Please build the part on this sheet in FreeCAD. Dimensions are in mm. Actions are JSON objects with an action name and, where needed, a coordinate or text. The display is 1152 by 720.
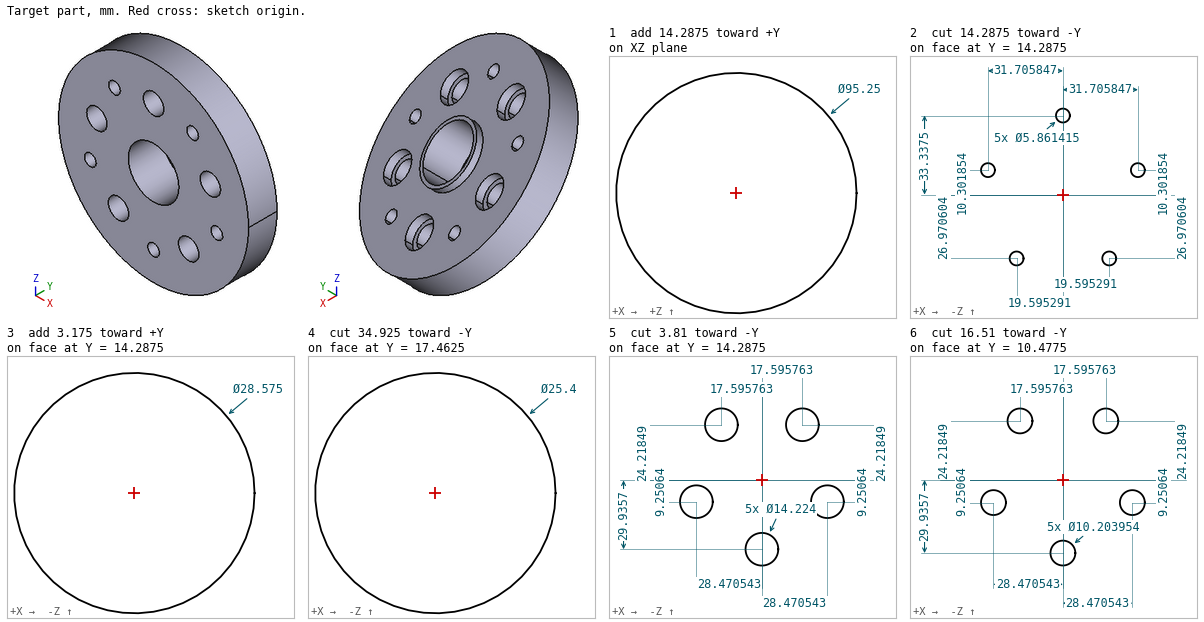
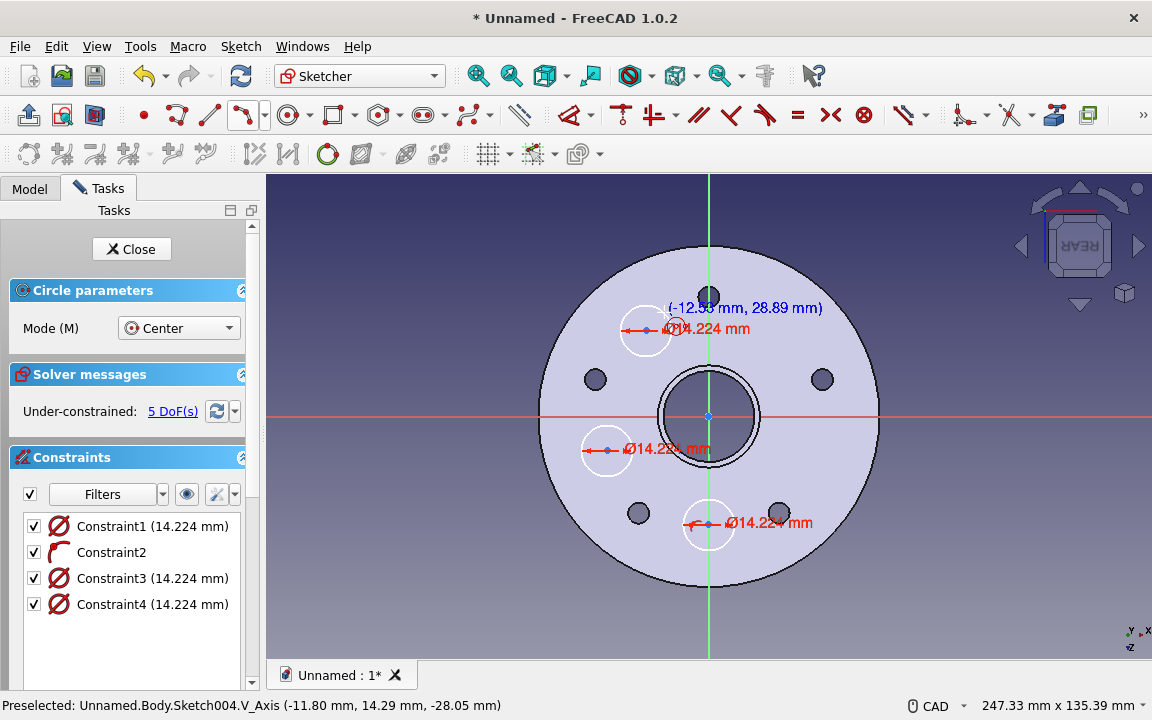
{"action": "left_click", "coordinate": [772, 330]}
{"action": "mouse_move", "coordinate": [790, 312]}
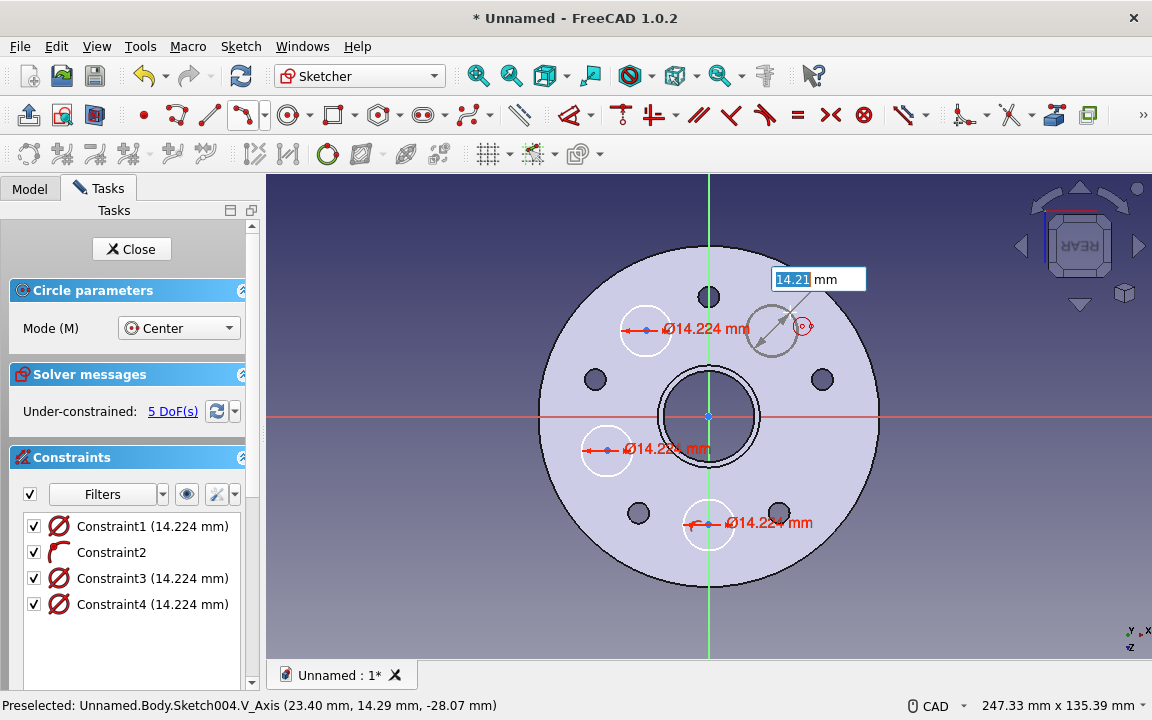
{"action": "type", "text": "14.224"}
{"action": "key", "text": "Return"}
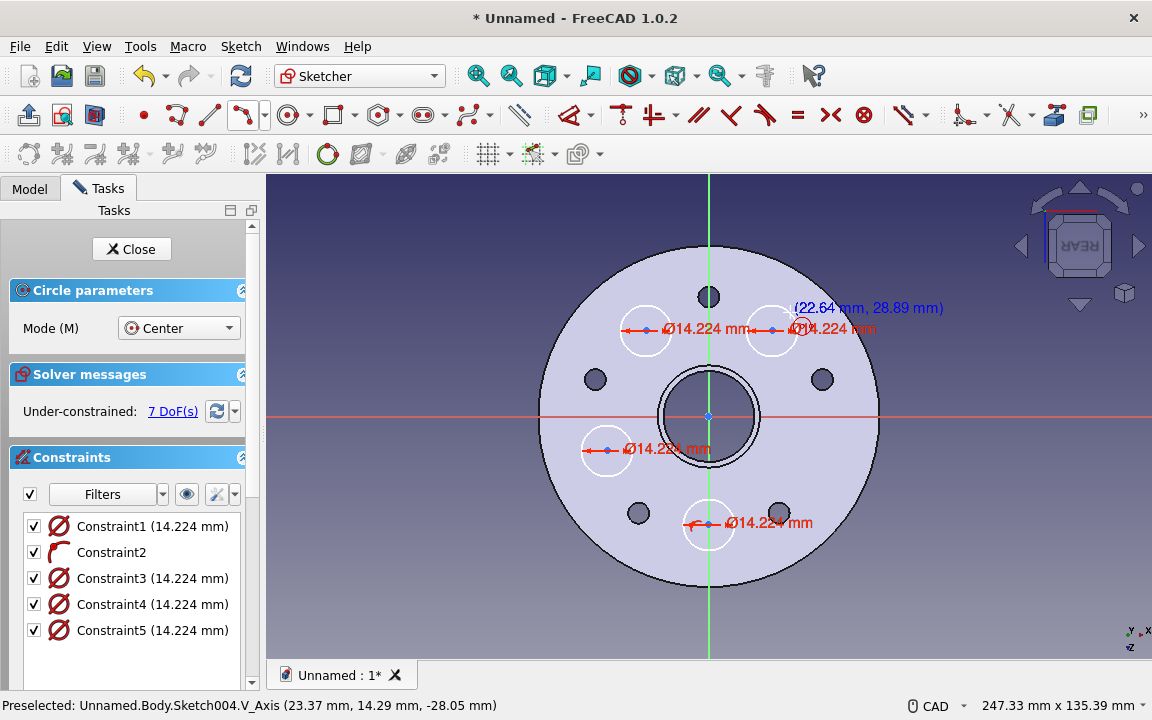
{"action": "left_click", "coordinate": [811, 450]}
{"action": "mouse_move", "coordinate": [829, 432]}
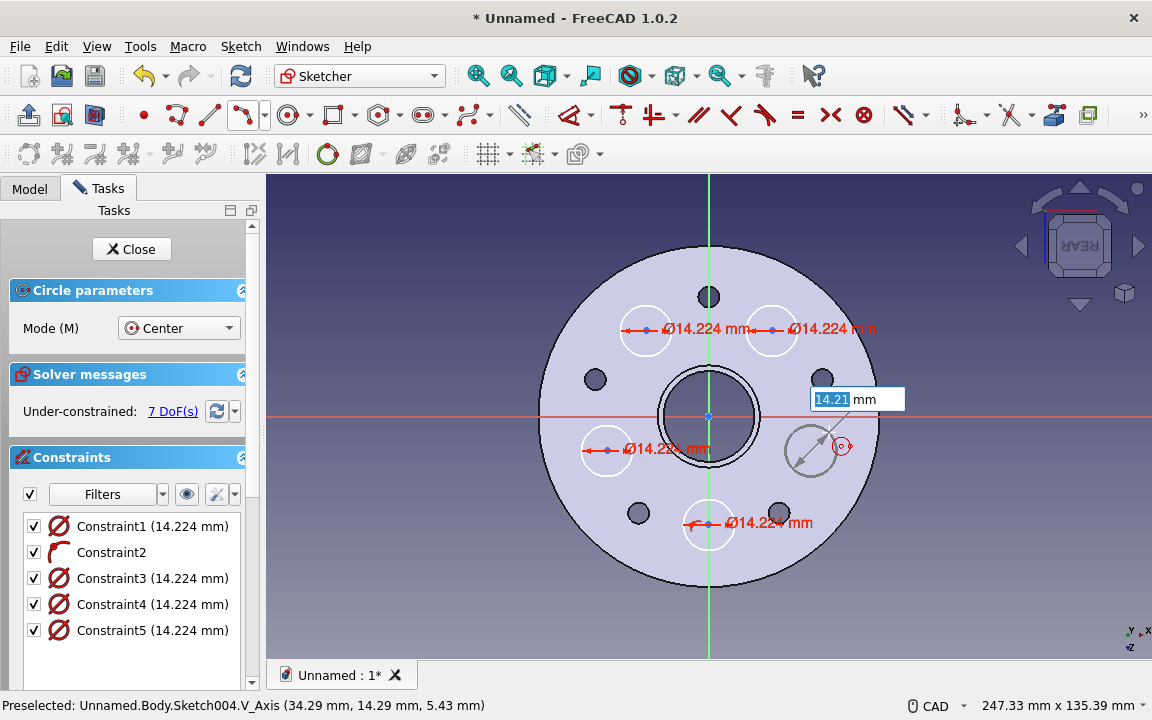
{"action": "type", "text": "14.224"}
{"action": "key", "text": "Return"}
{"action": "key", "text": "Escape"}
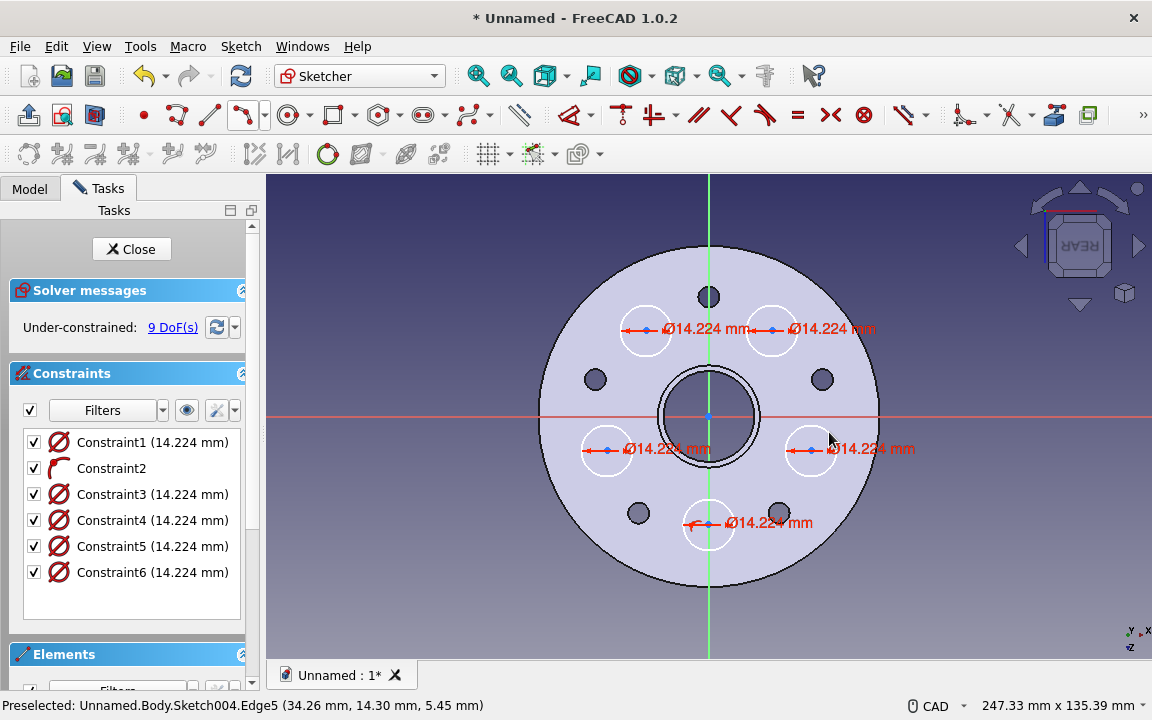
{"action": "left_click", "coordinate": [568, 116]}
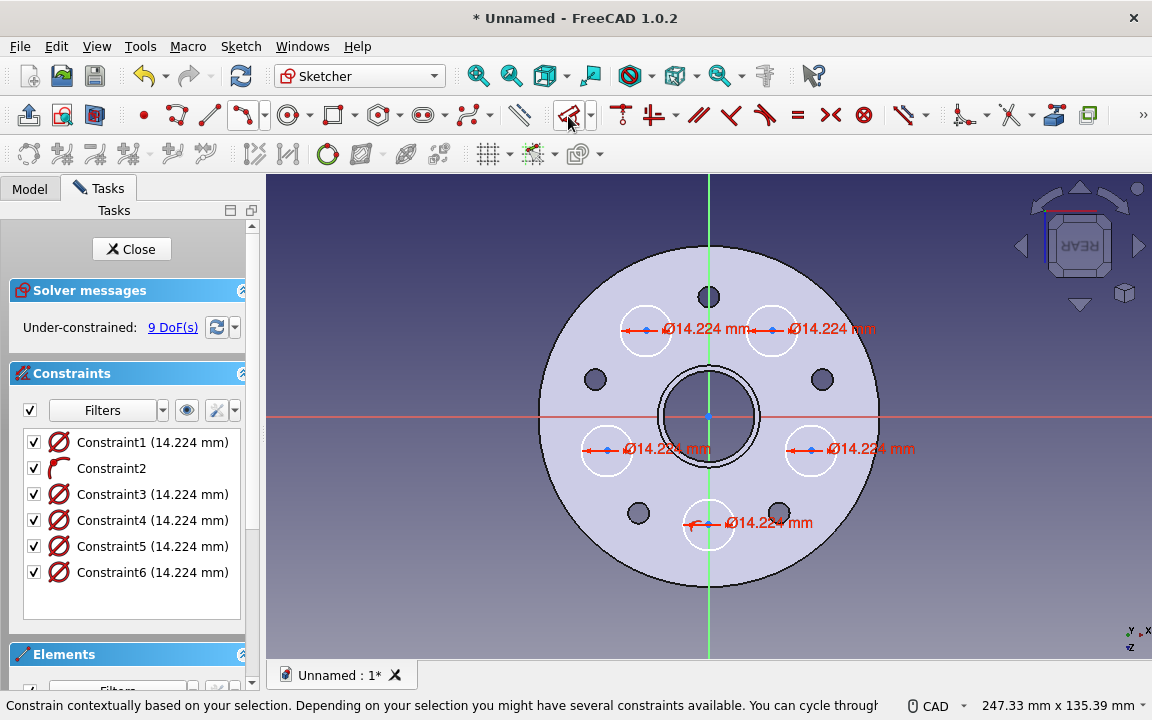
{"action": "left_click", "coordinate": [709, 525]}
{"action": "left_click", "coordinate": [743, 471]}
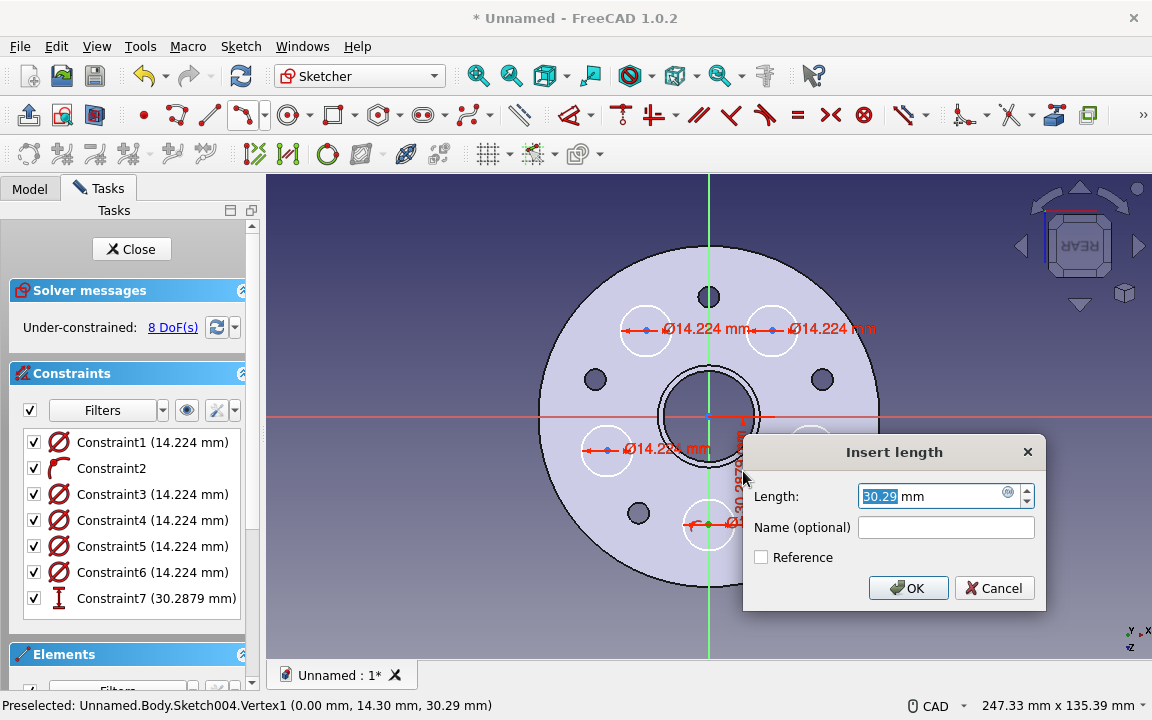
{"action": "type", "text": "29.9357"}
{"action": "key", "text": "Return"}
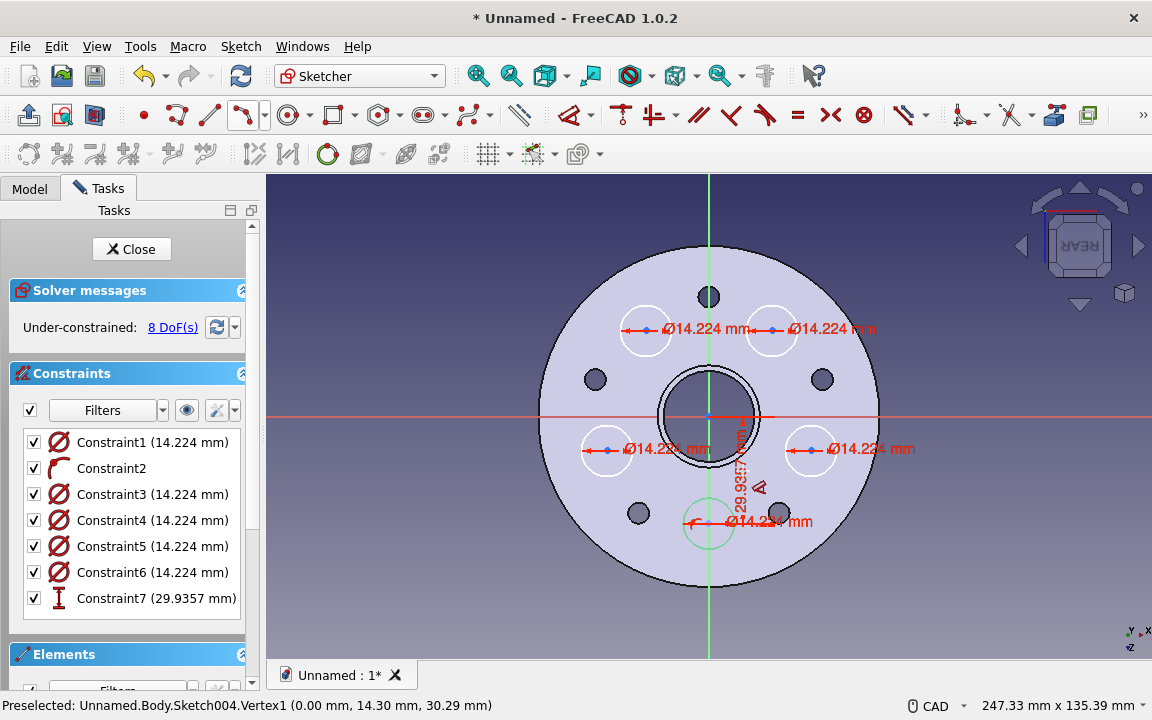
{"action": "left_click", "coordinate": [607, 451]}
{"action": "left_click", "coordinate": [743, 434]}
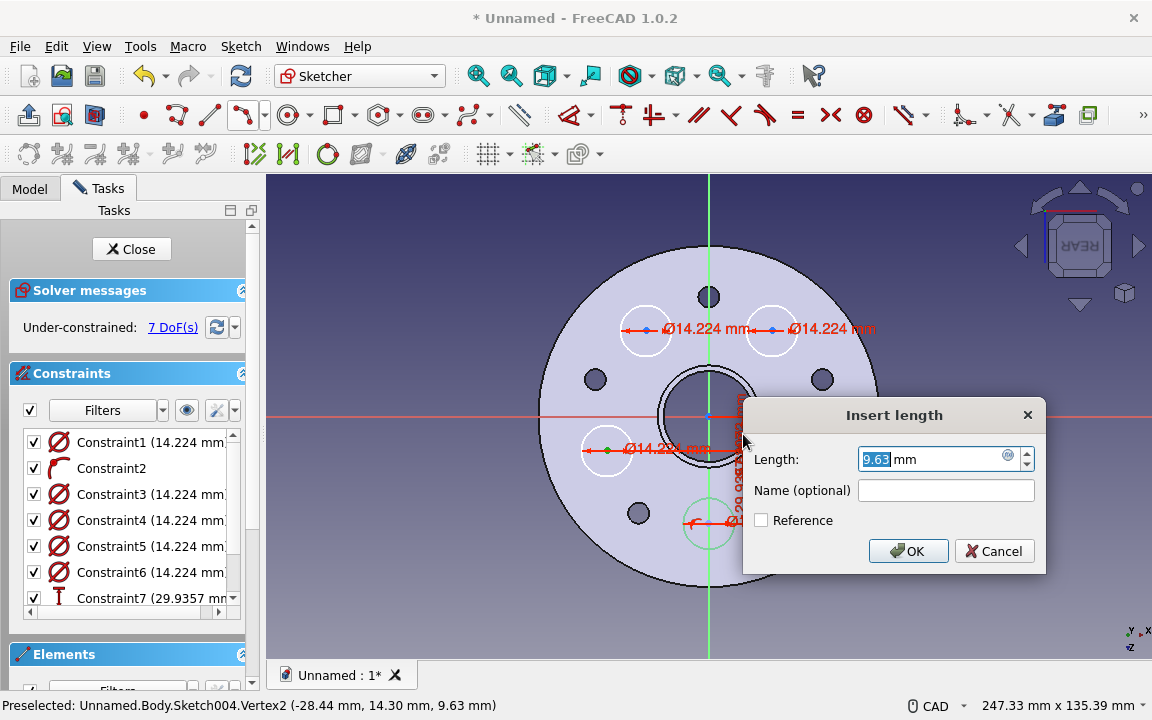
{"action": "type", "text": "9.25064"}
{"action": "key", "text": "Return"}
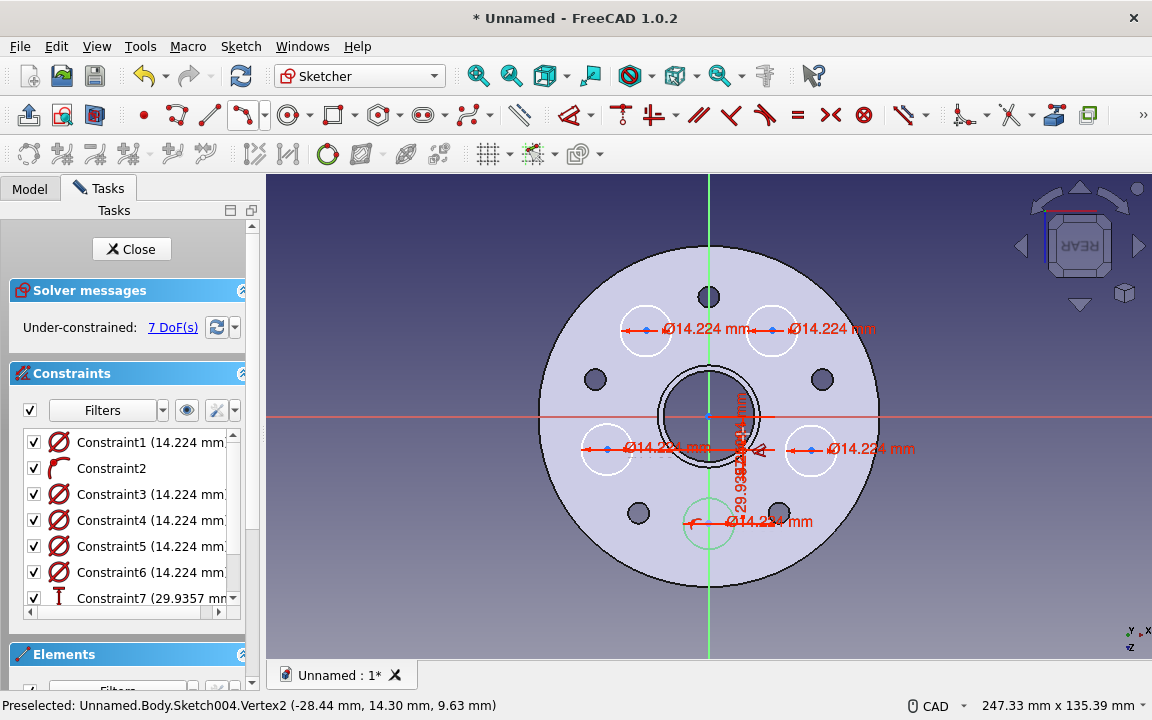
{"action": "left_click", "coordinate": [811, 451]}
{"action": "left_click", "coordinate": [869, 434]}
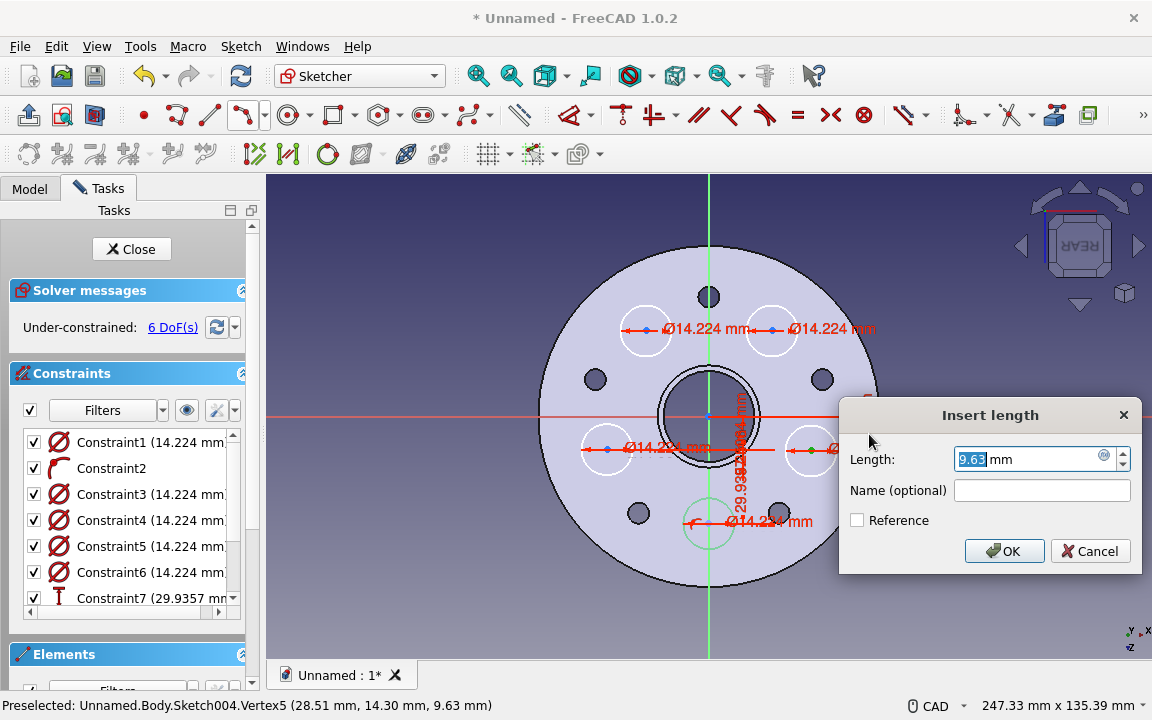
{"action": "type", "text": "9.25064"}
{"action": "key", "text": "Return"}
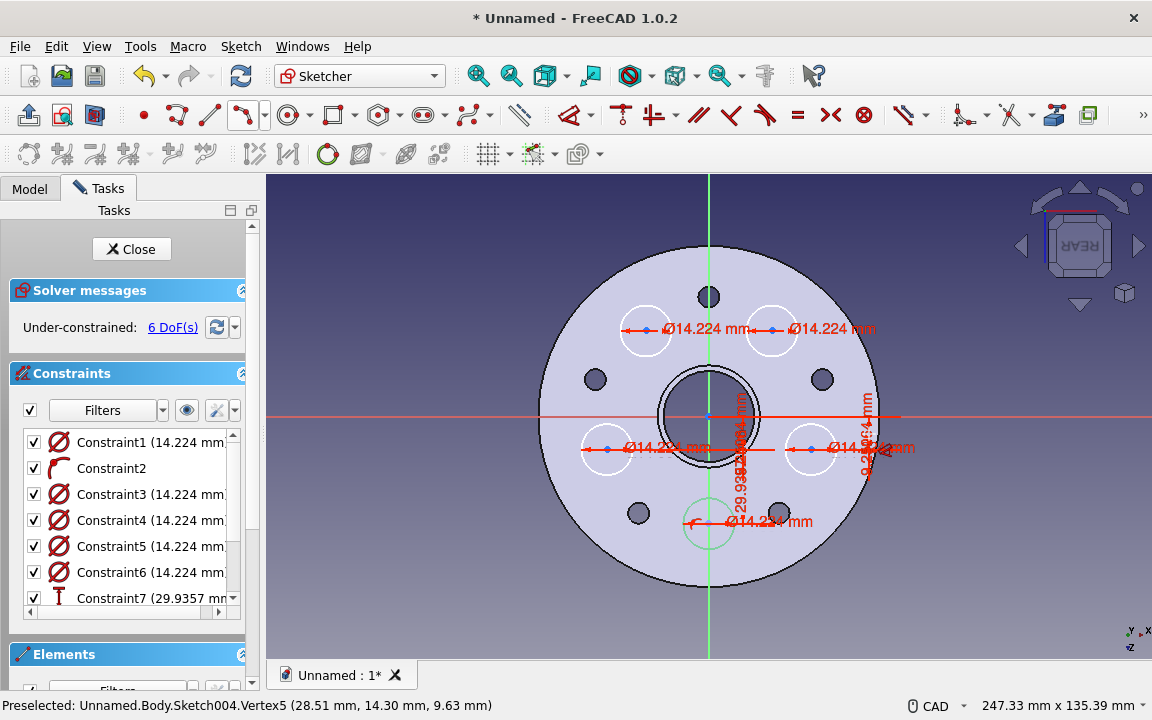
{"action": "left_click", "coordinate": [646, 331]}
{"action": "left_click", "coordinate": [612, 374]}